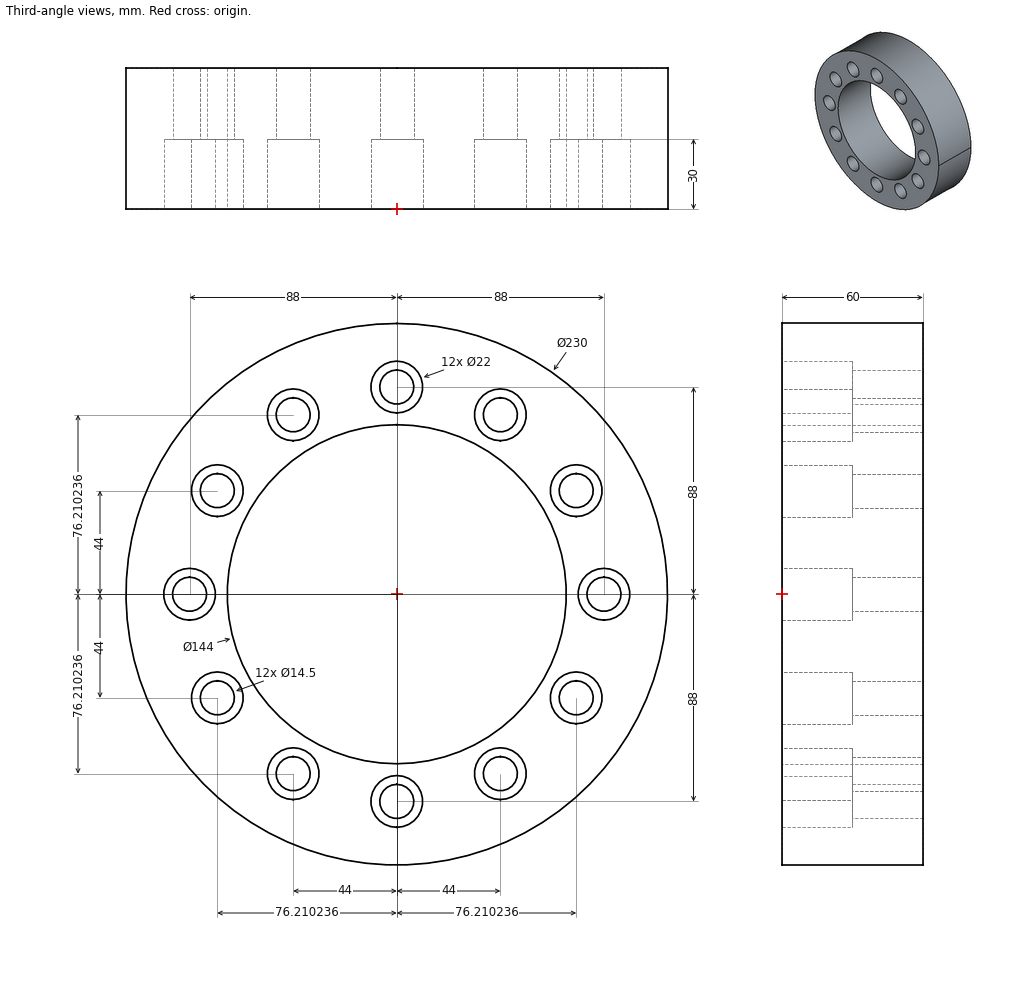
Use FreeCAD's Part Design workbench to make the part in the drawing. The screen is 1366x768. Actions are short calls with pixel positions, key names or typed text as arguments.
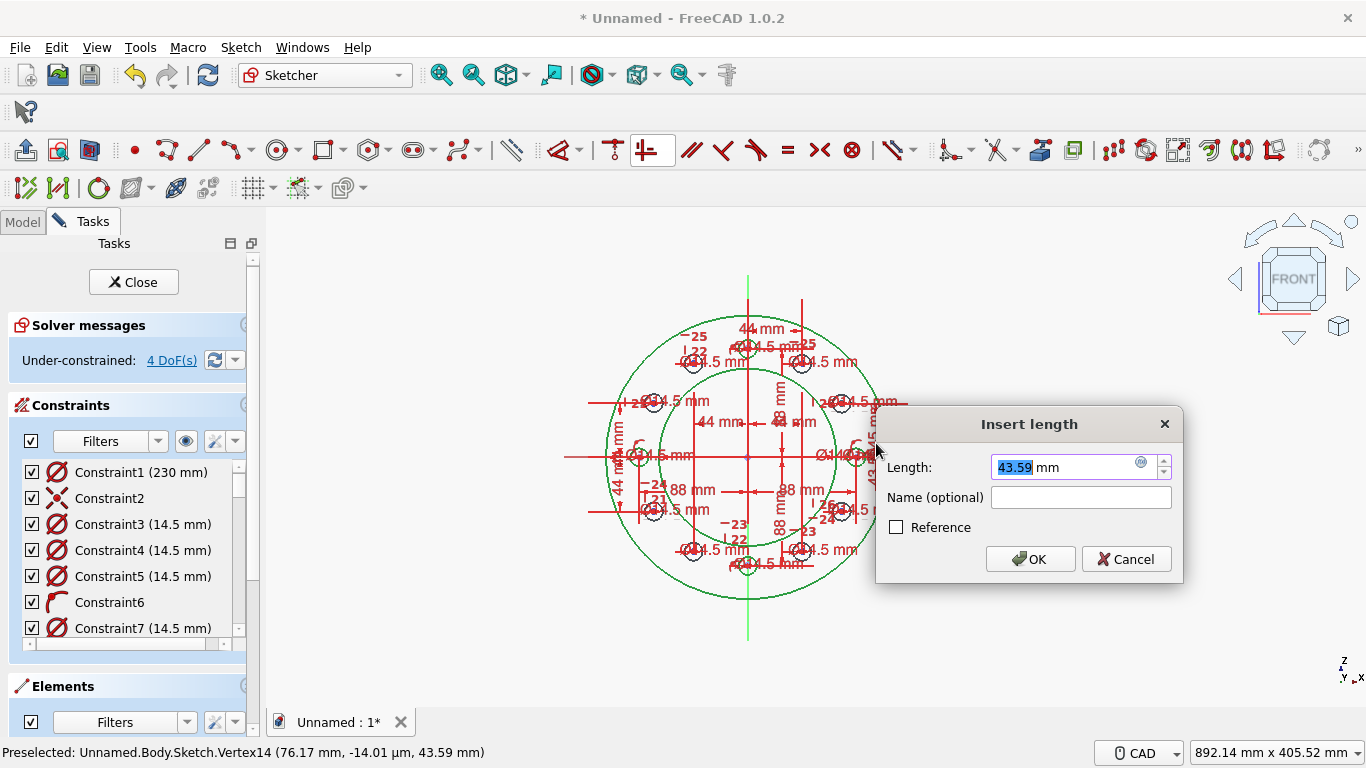
text(44)
key(Return)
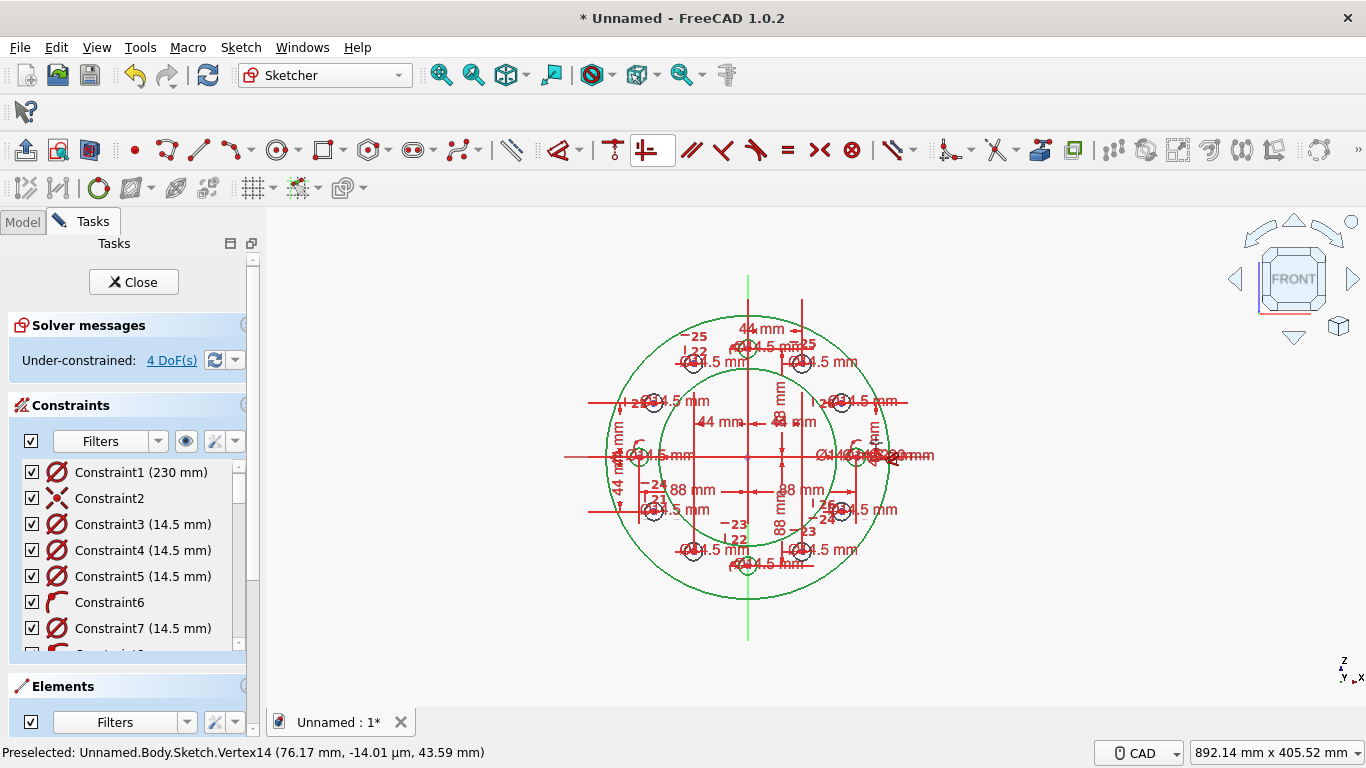
click(654, 512)
click(668, 546)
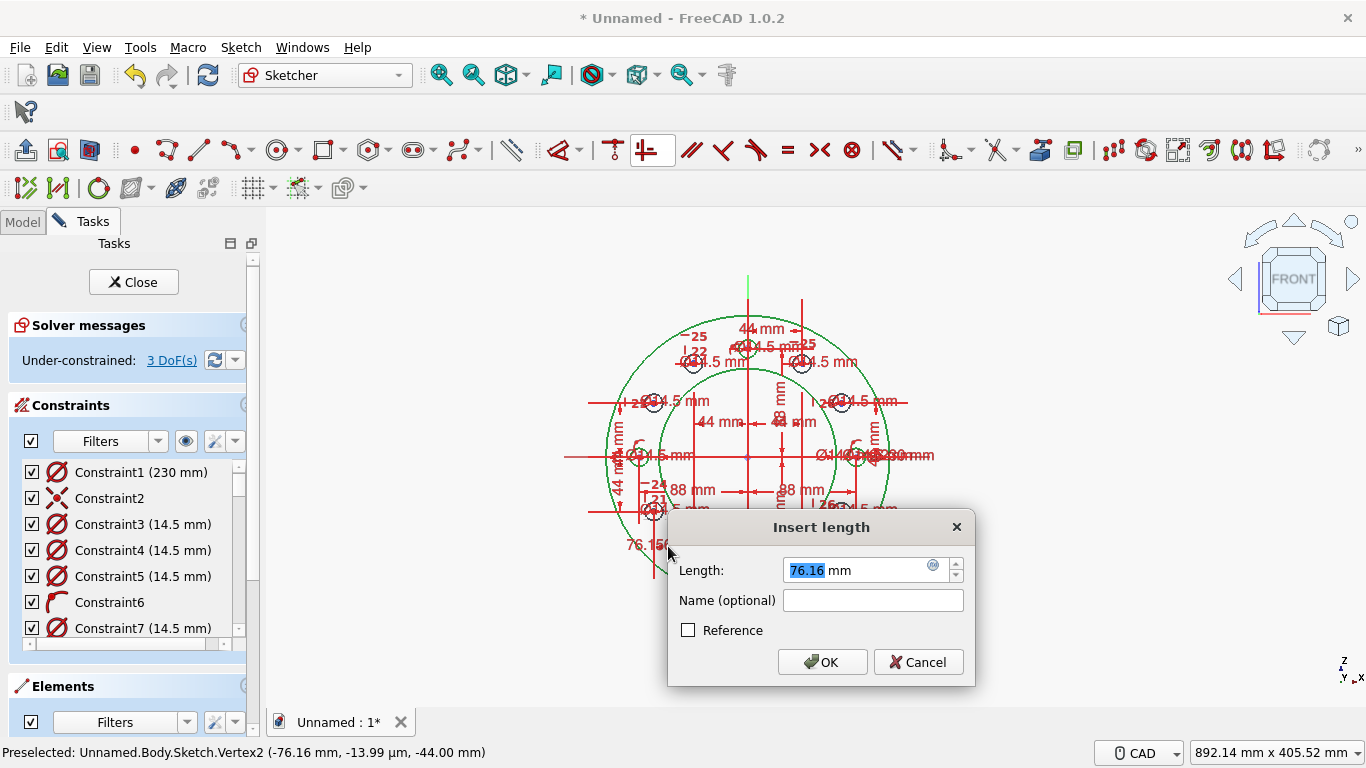
text(76.210236)
key(Return)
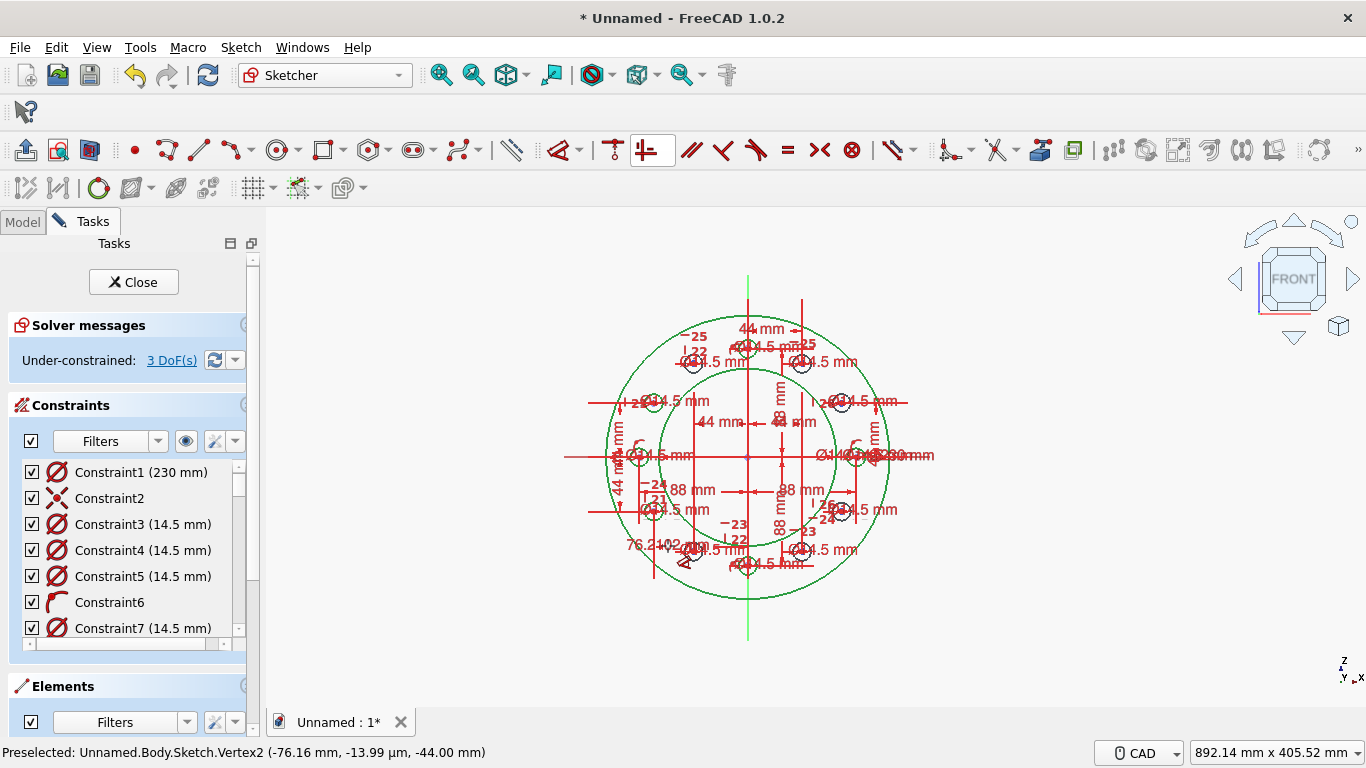
click(694, 552)
click(830, 538)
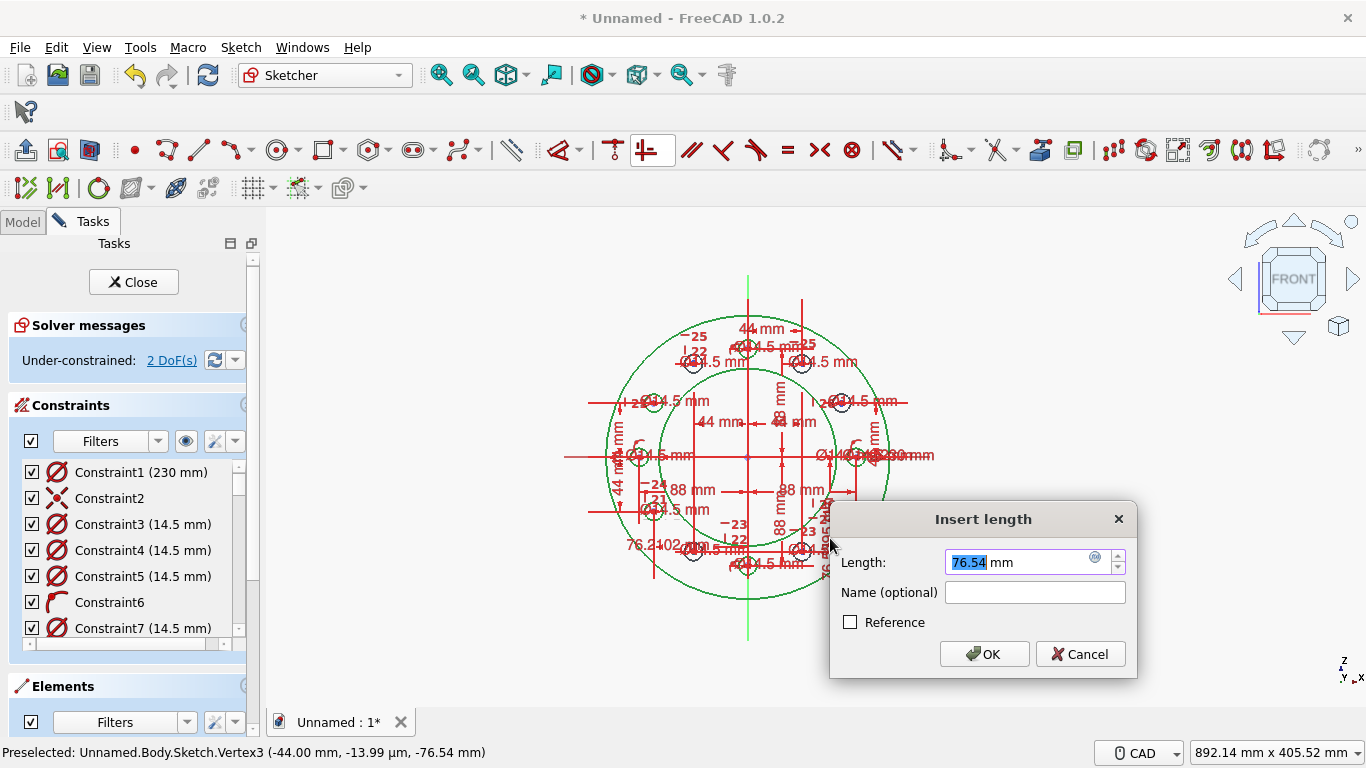
text(76.210236)
key(Return)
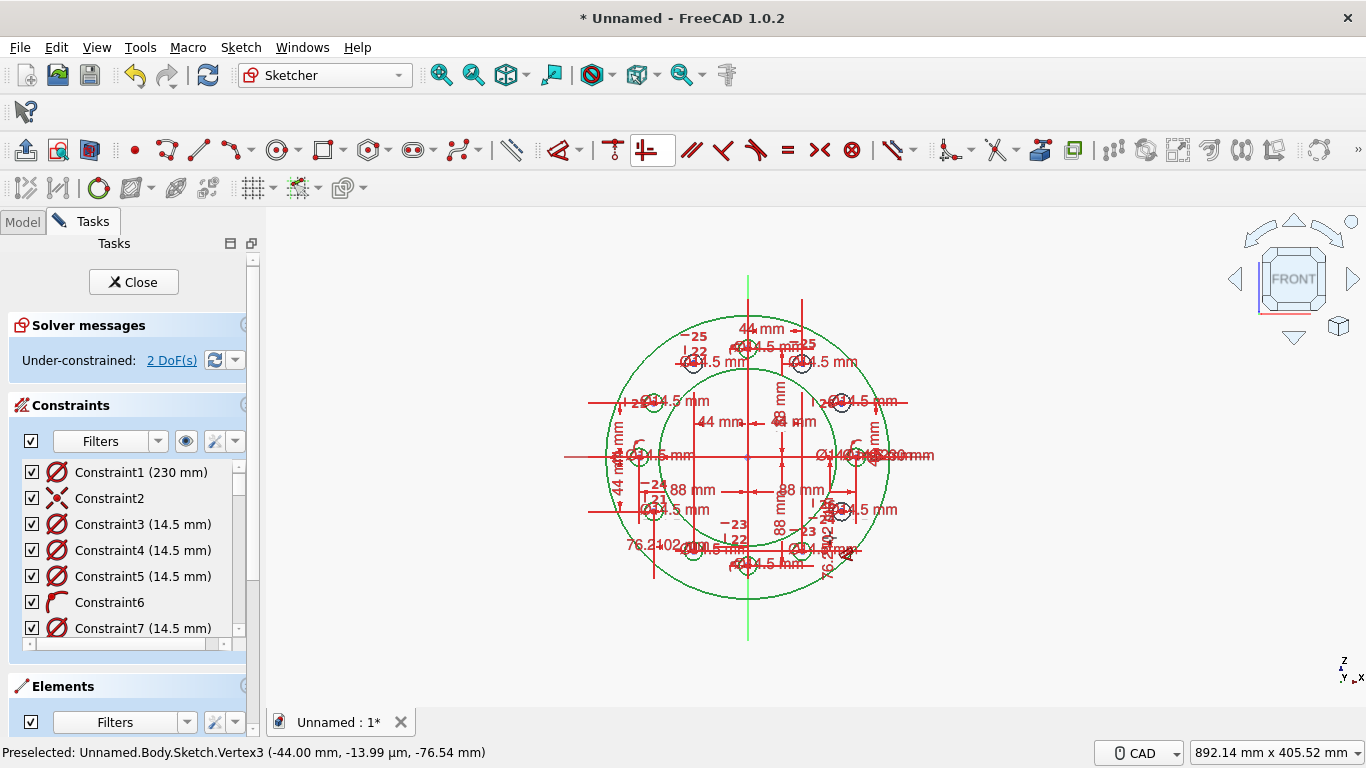
click(694, 364)
click(660, 378)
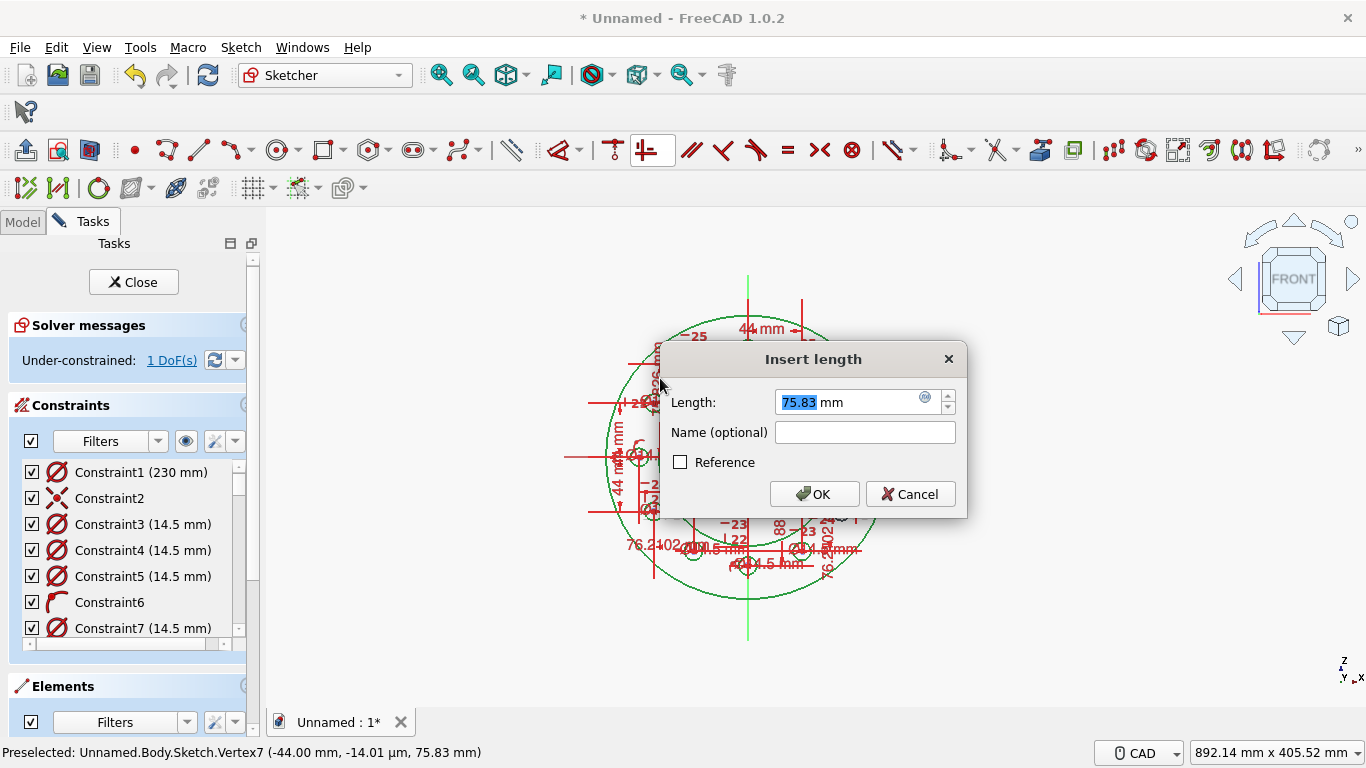
text(76.210236)
key(Return)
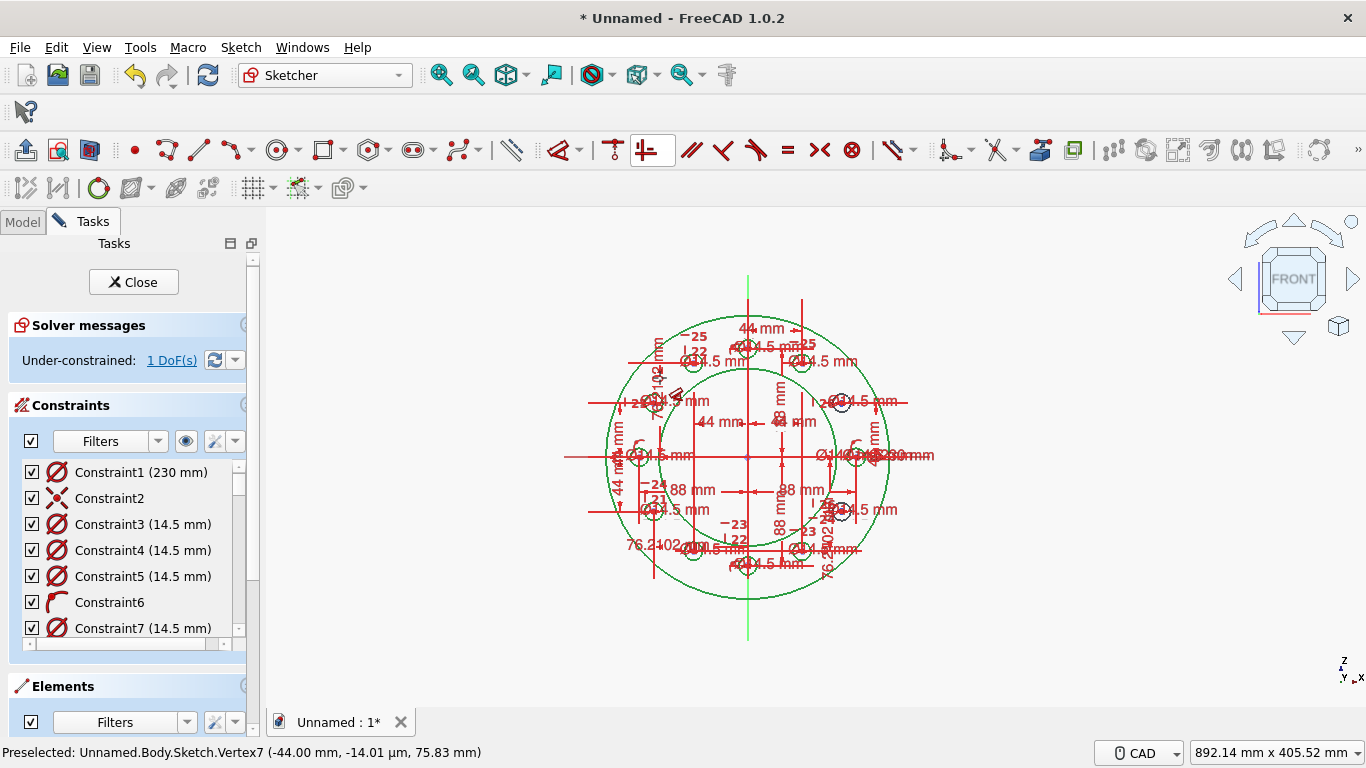
click(842, 512)
click(773, 570)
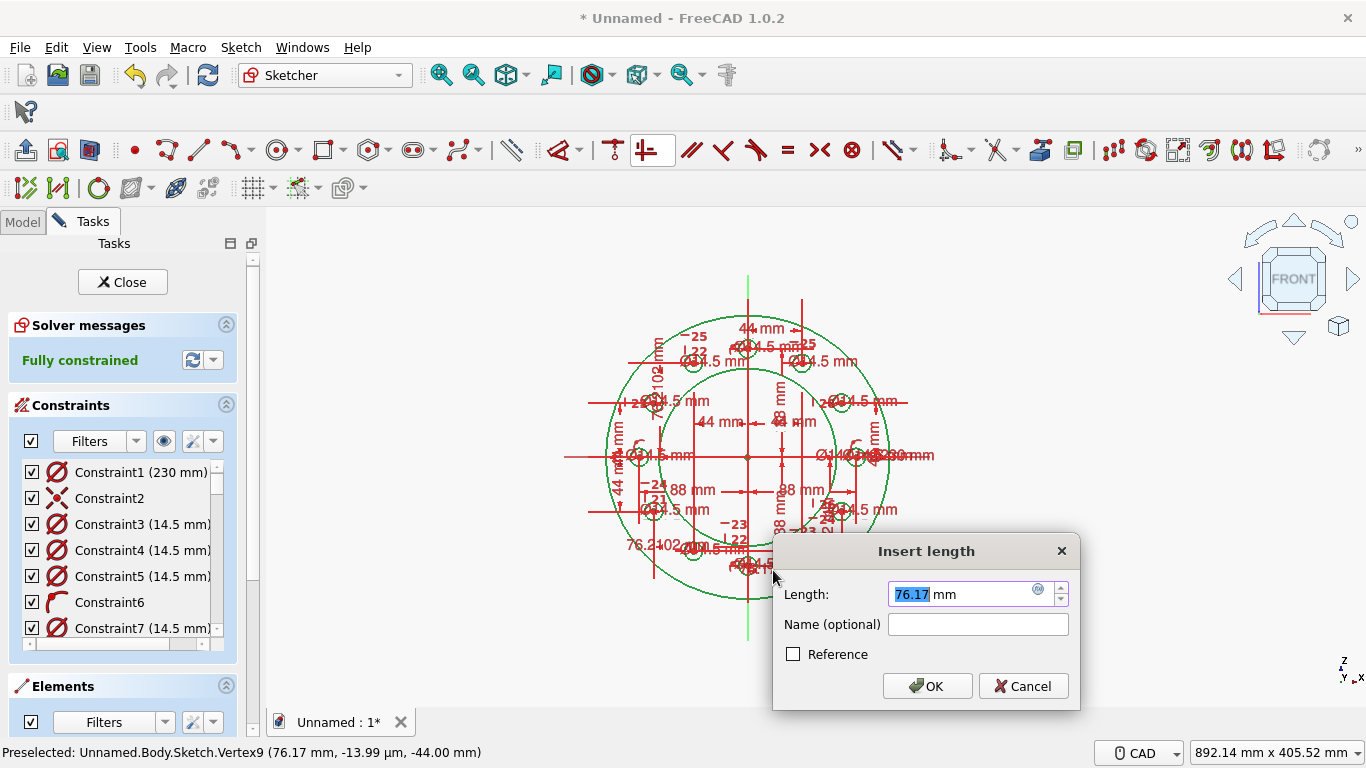
text(76.210236)
key(Return)
key(Escape)